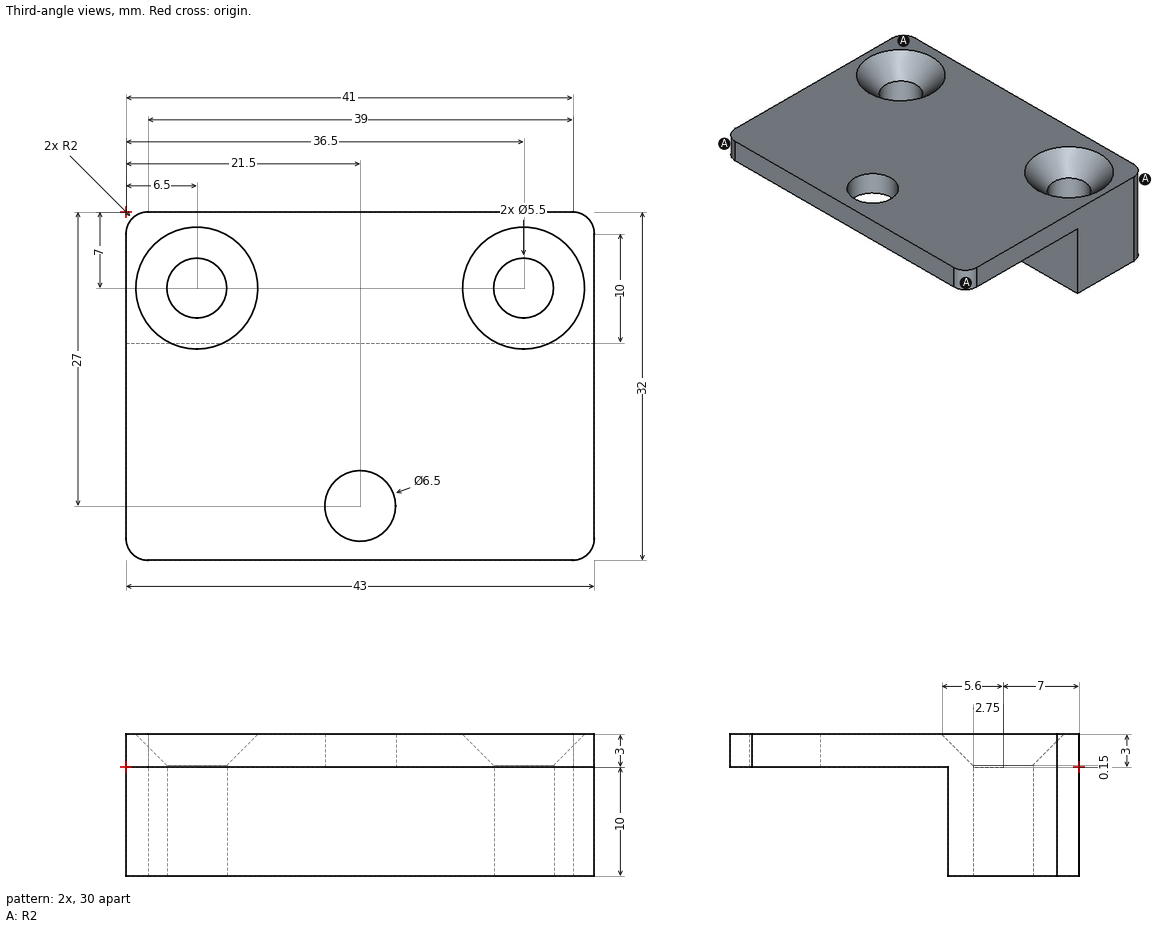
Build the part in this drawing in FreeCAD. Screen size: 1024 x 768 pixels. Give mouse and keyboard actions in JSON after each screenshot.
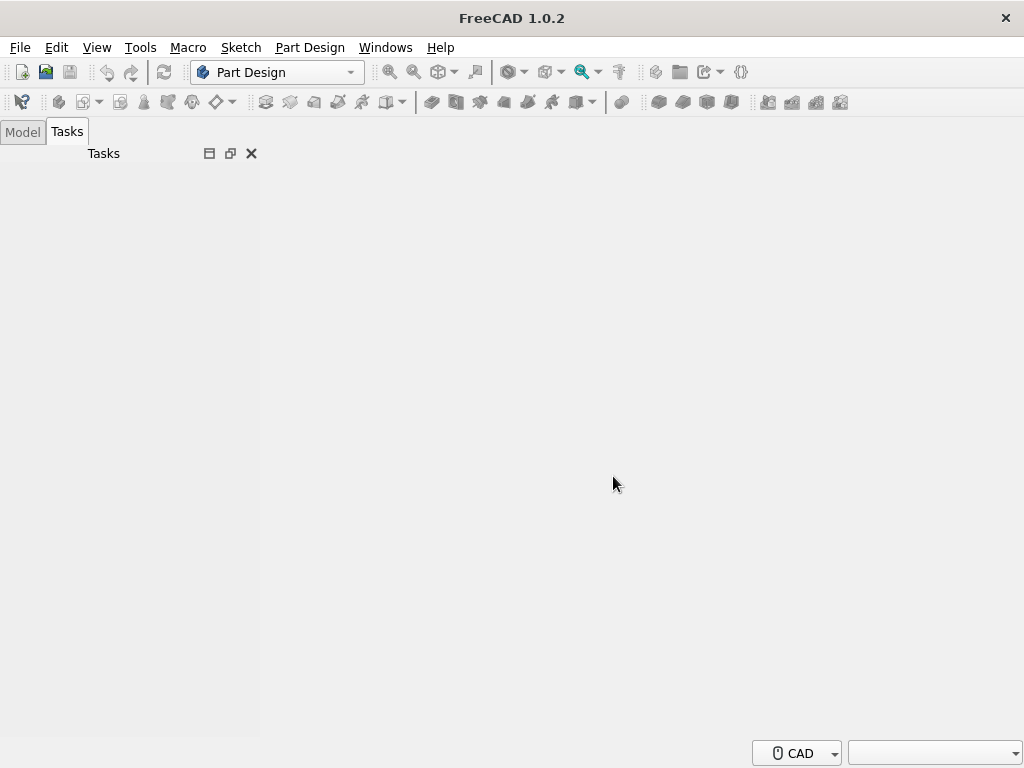
{"action": "key", "text": "ctrl+n"}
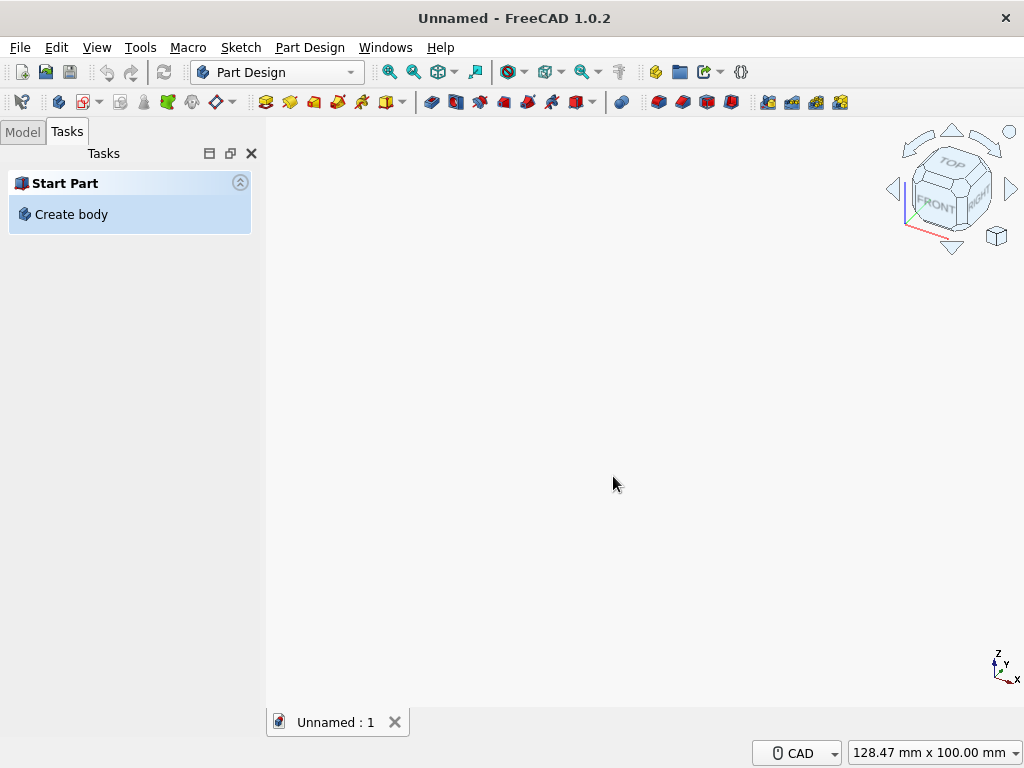
{"action": "left_click", "coordinate": [84, 102]}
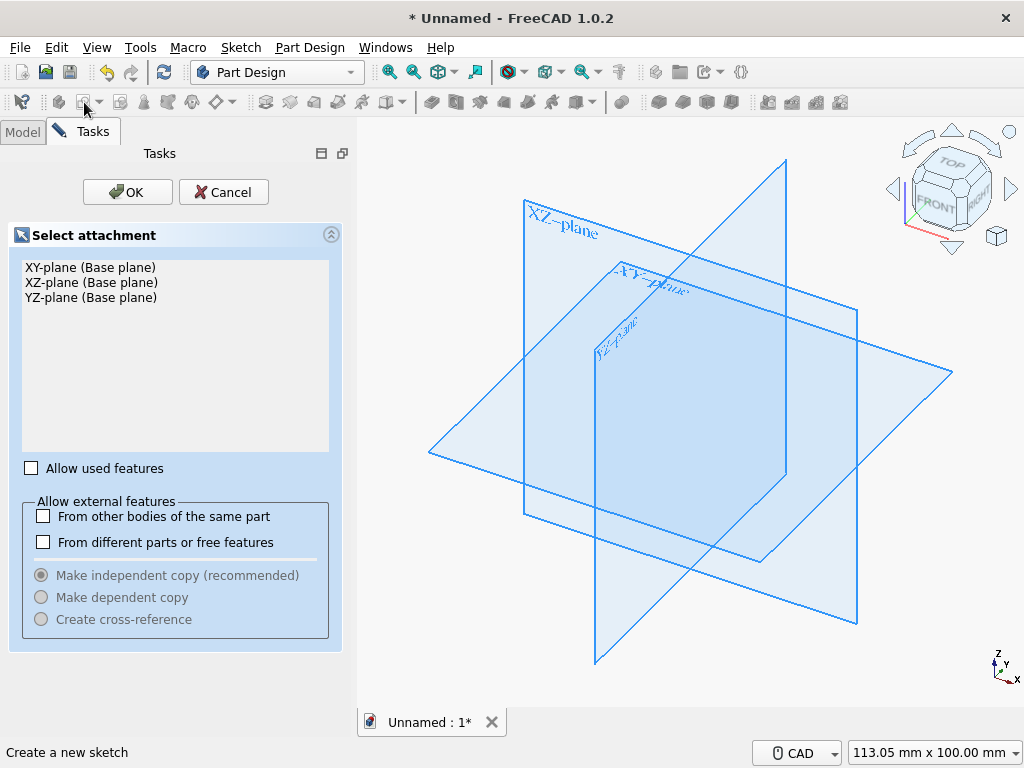
{"action": "left_click", "coordinate": [82, 268]}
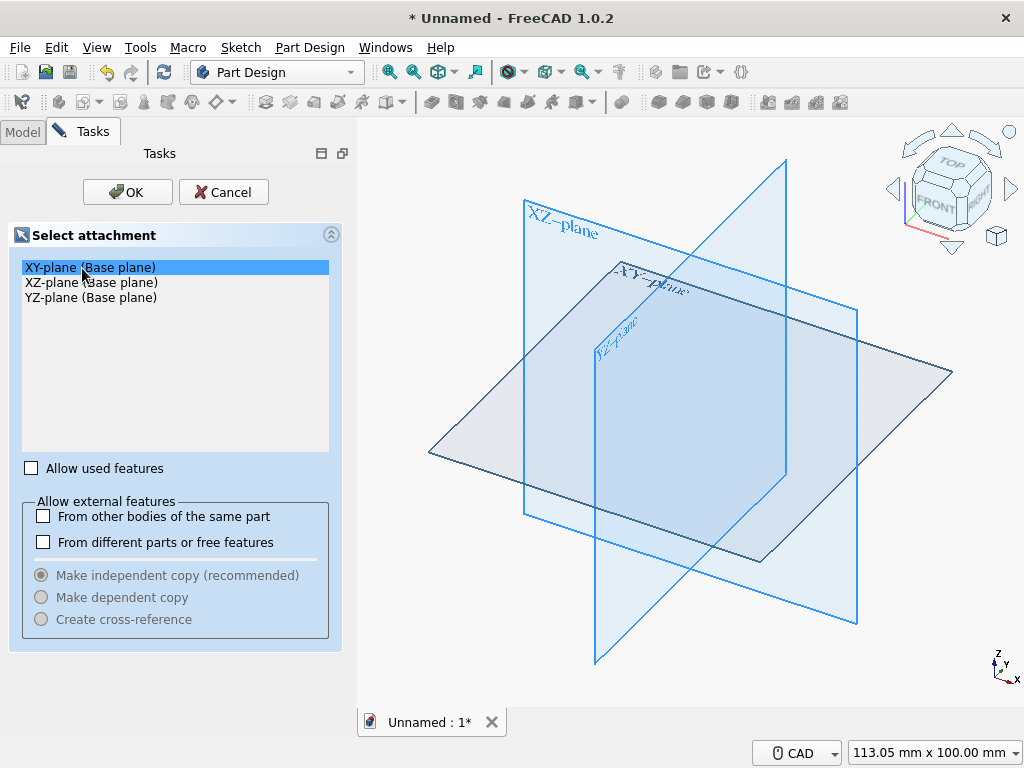
{"action": "left_click", "coordinate": [128, 192]}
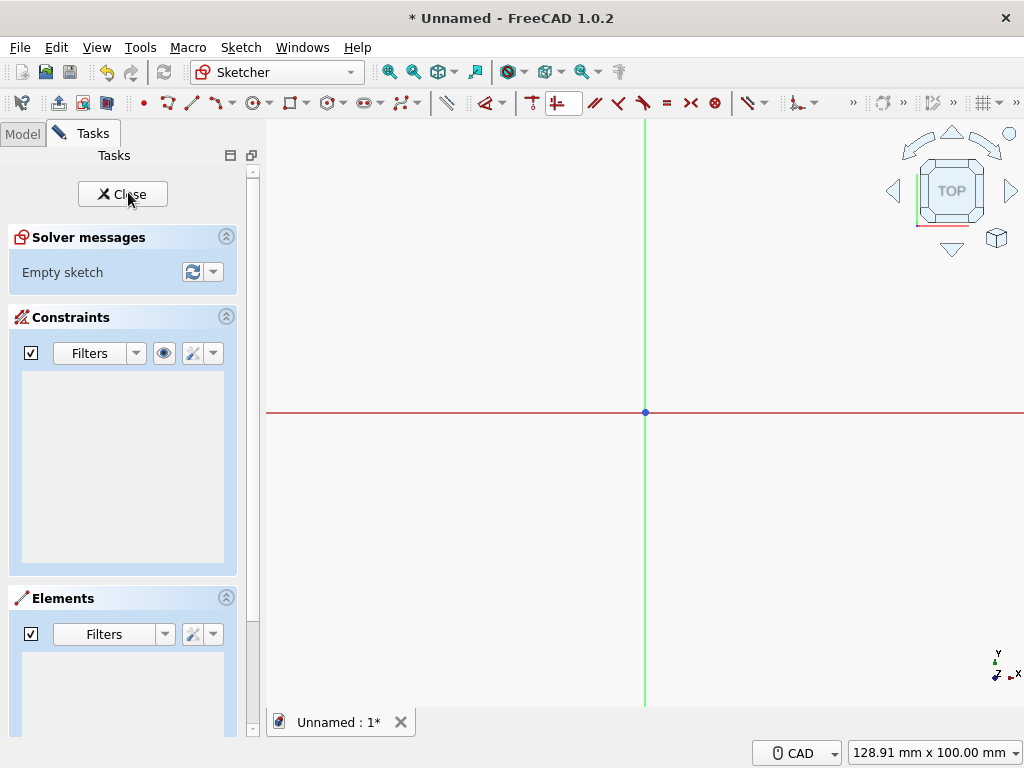
{"action": "scroll", "coordinate": [294, 147], "scroll_direction": "down", "scroll_amount": 1}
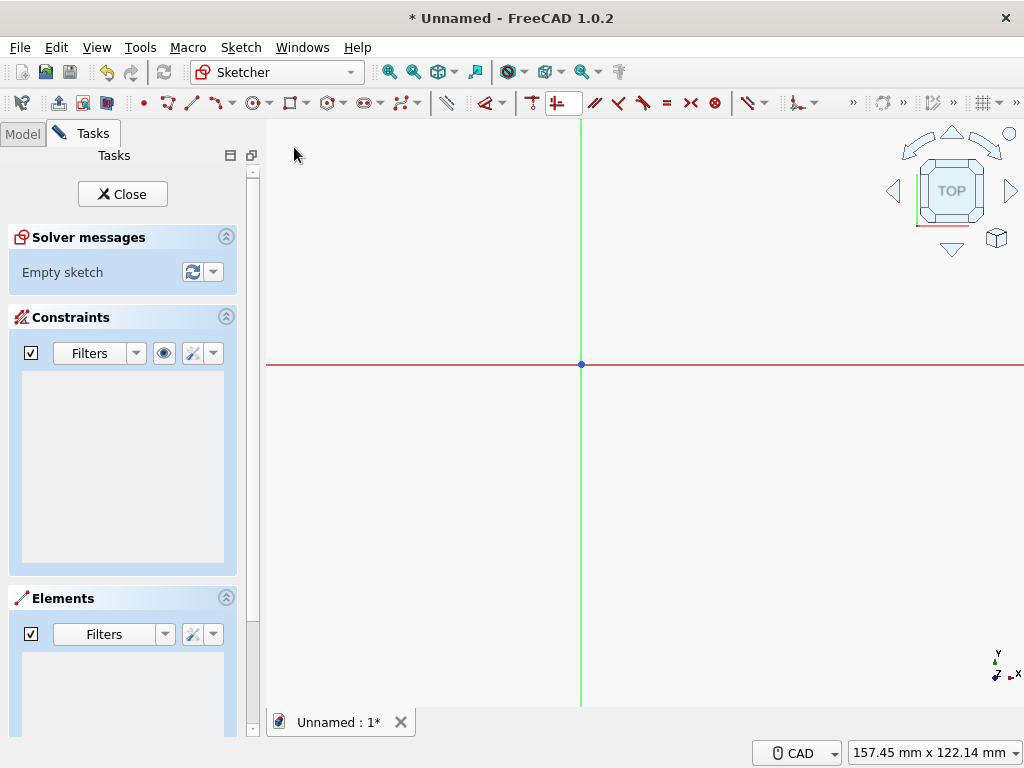
{"action": "scroll", "coordinate": [817, 477], "scroll_direction": "up", "scroll_amount": 3}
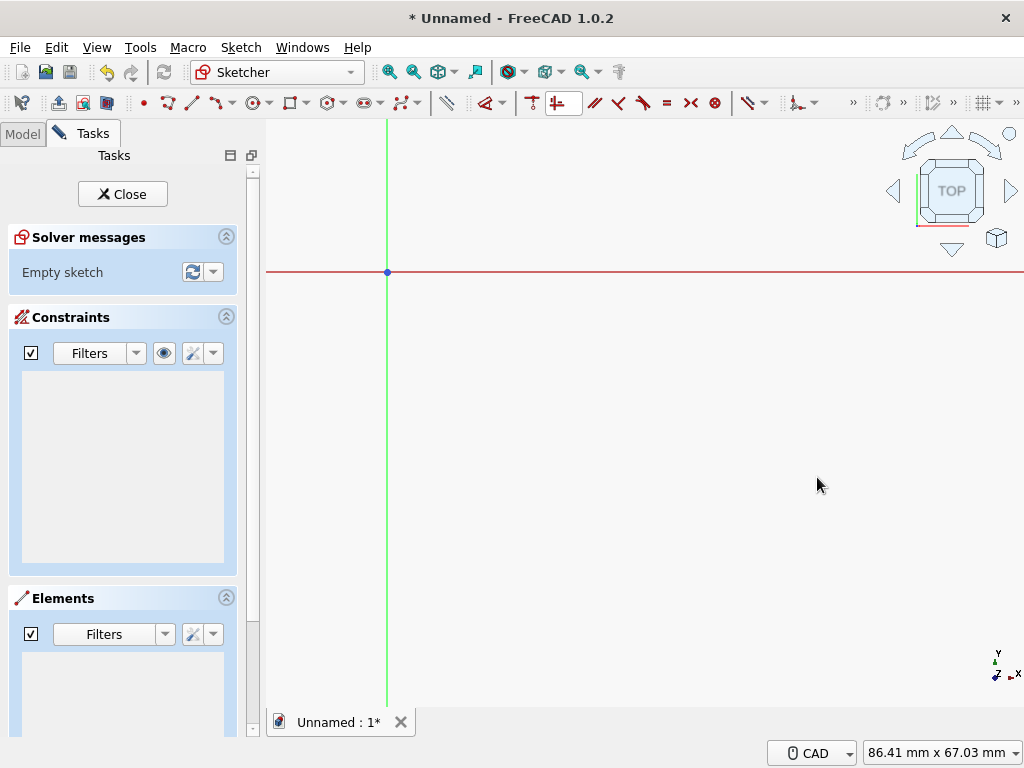
{"action": "key", "text": "g r"}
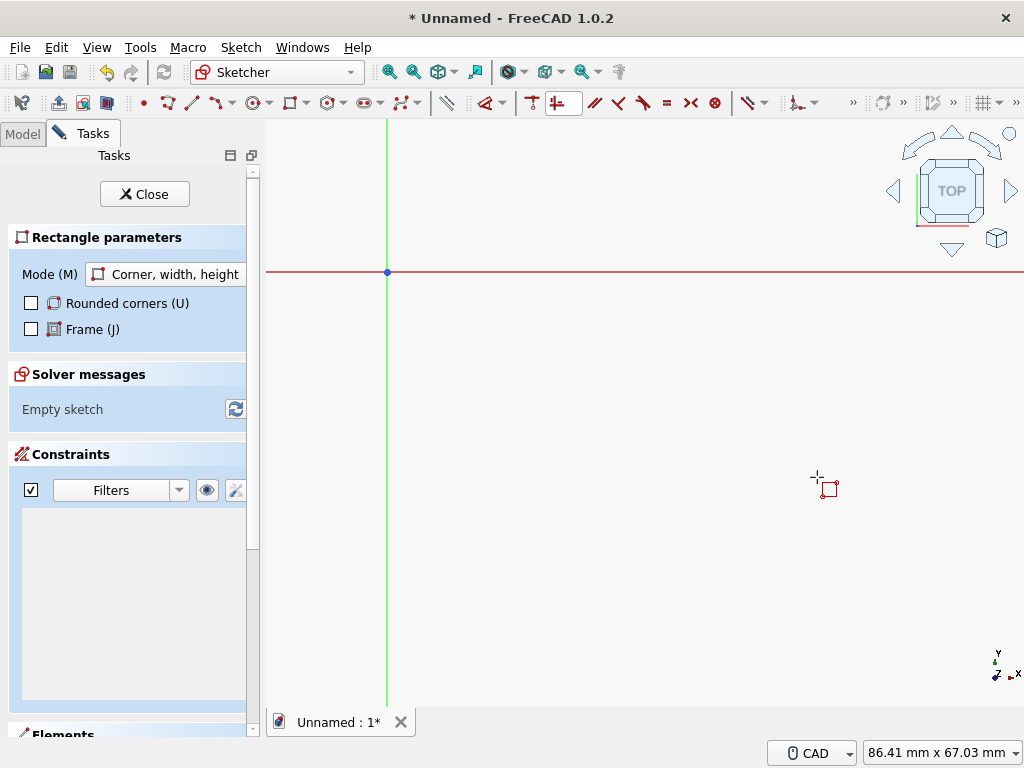
{"action": "left_click", "coordinate": [387, 272]}
{"action": "mouse_move", "coordinate": [764, 553]}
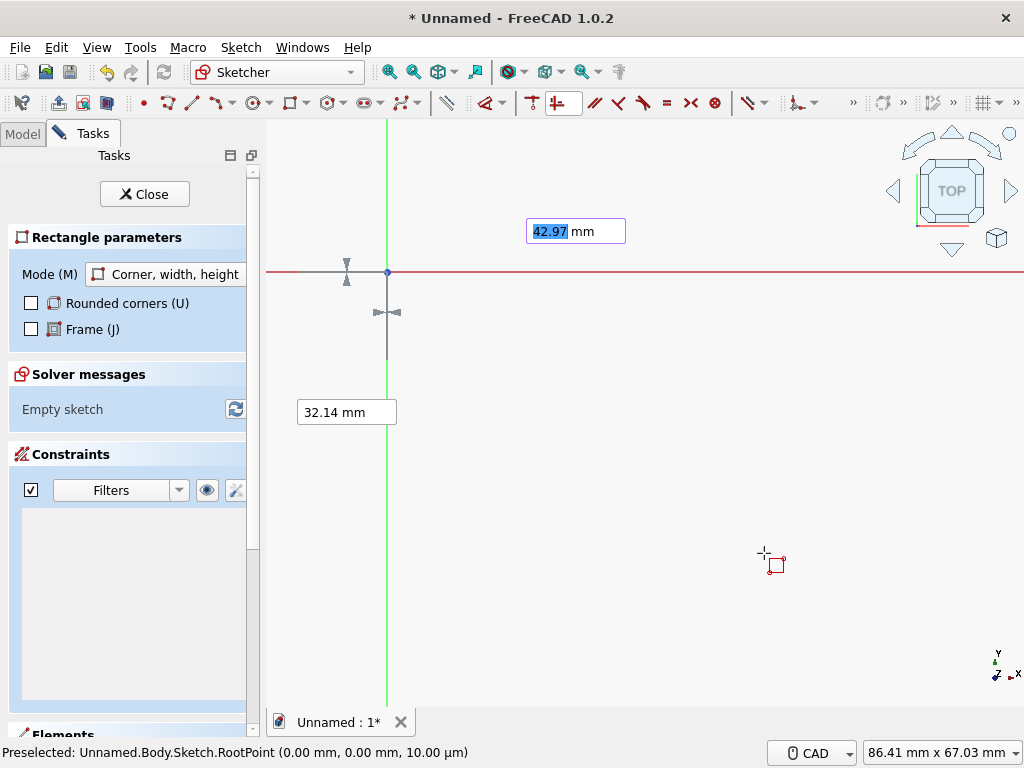
{"action": "type", "text": "43"}
{"action": "key", "text": "Tab"}
{"action": "type", "text": "32"}
{"action": "key", "text": "Return"}
{"action": "key", "text": "Escape"}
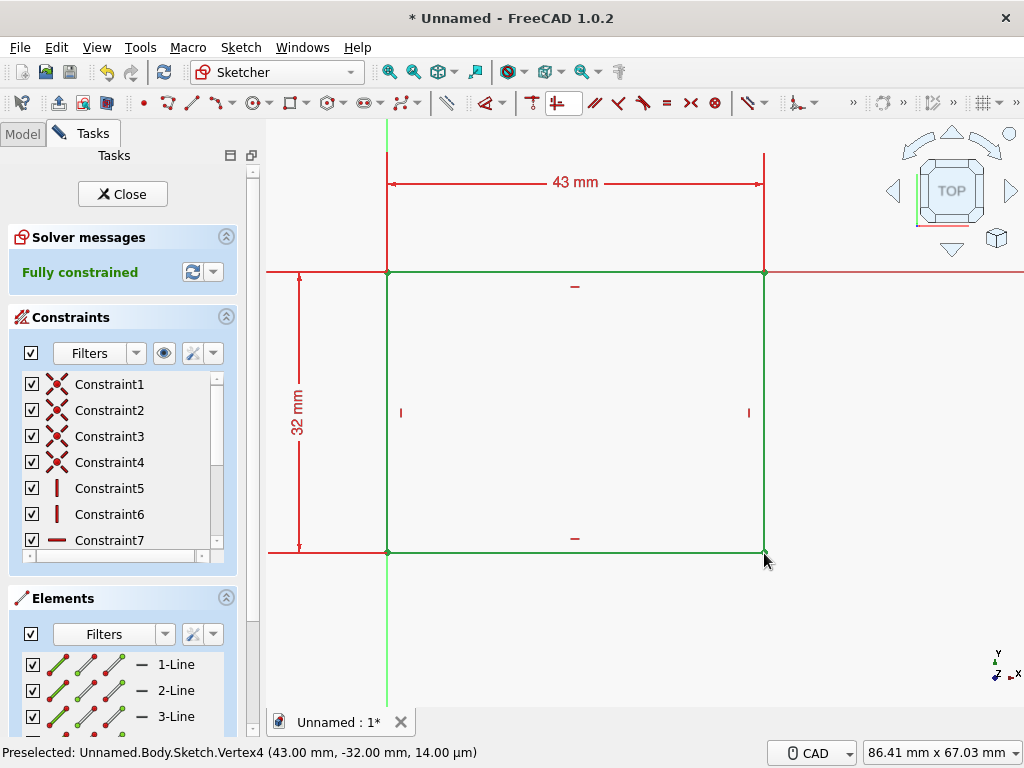
{"action": "left_click", "coordinate": [123, 194]}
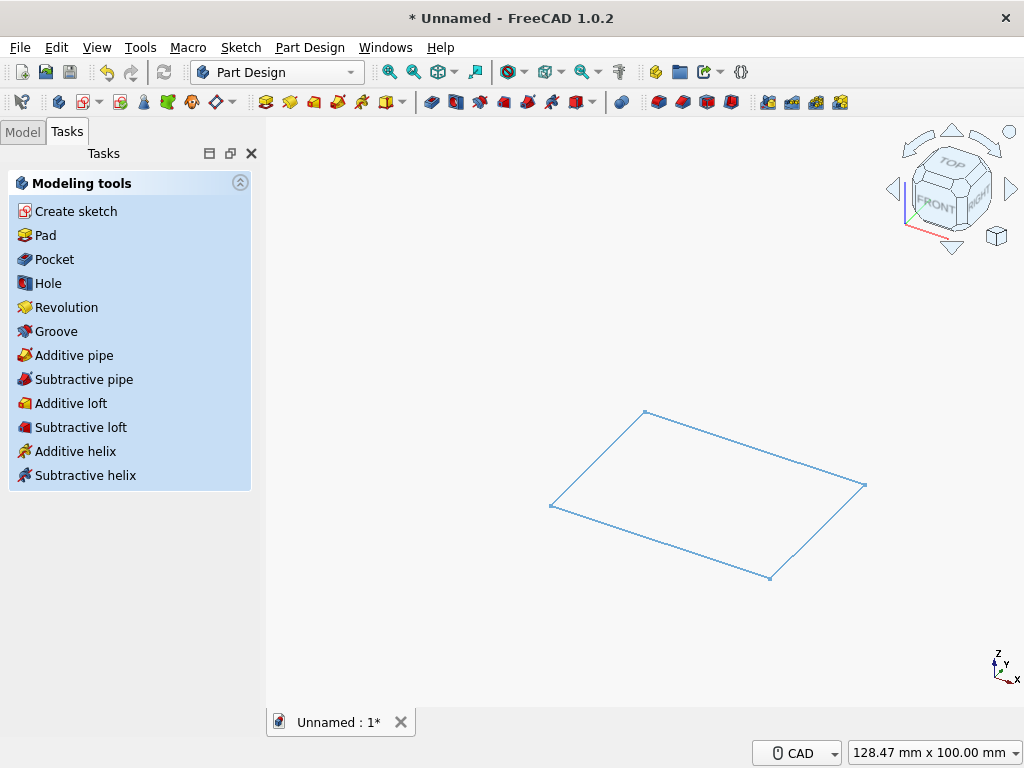
{"action": "left_click", "coordinate": [266, 102]}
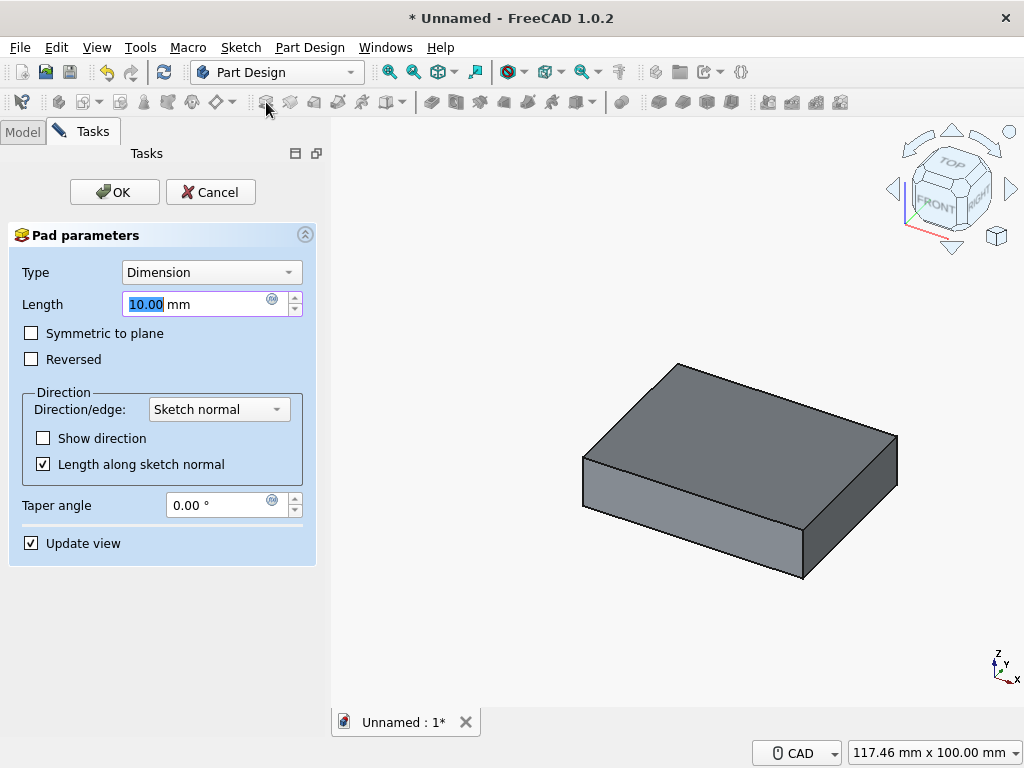
{"action": "type", "text": "3"}
{"action": "key", "text": "Tab"}